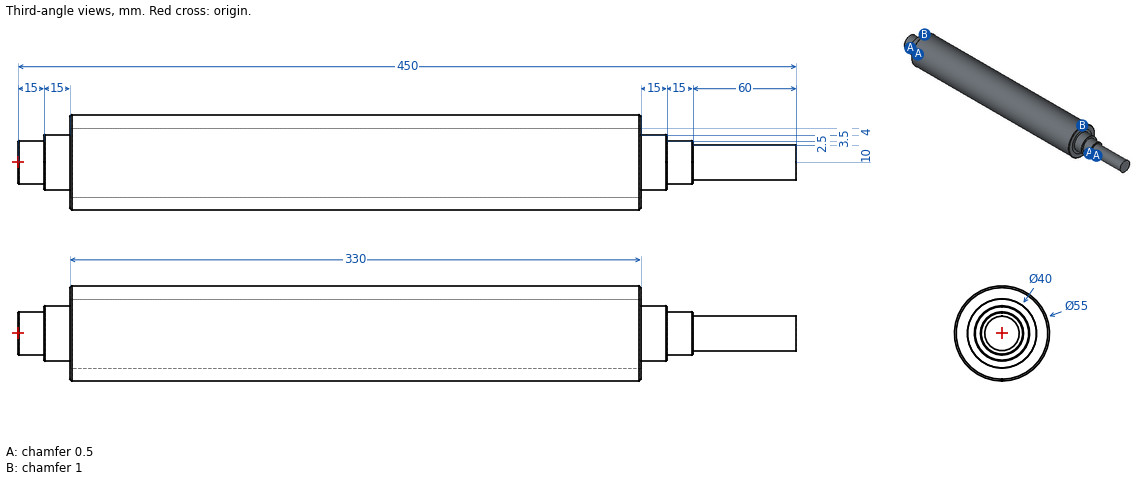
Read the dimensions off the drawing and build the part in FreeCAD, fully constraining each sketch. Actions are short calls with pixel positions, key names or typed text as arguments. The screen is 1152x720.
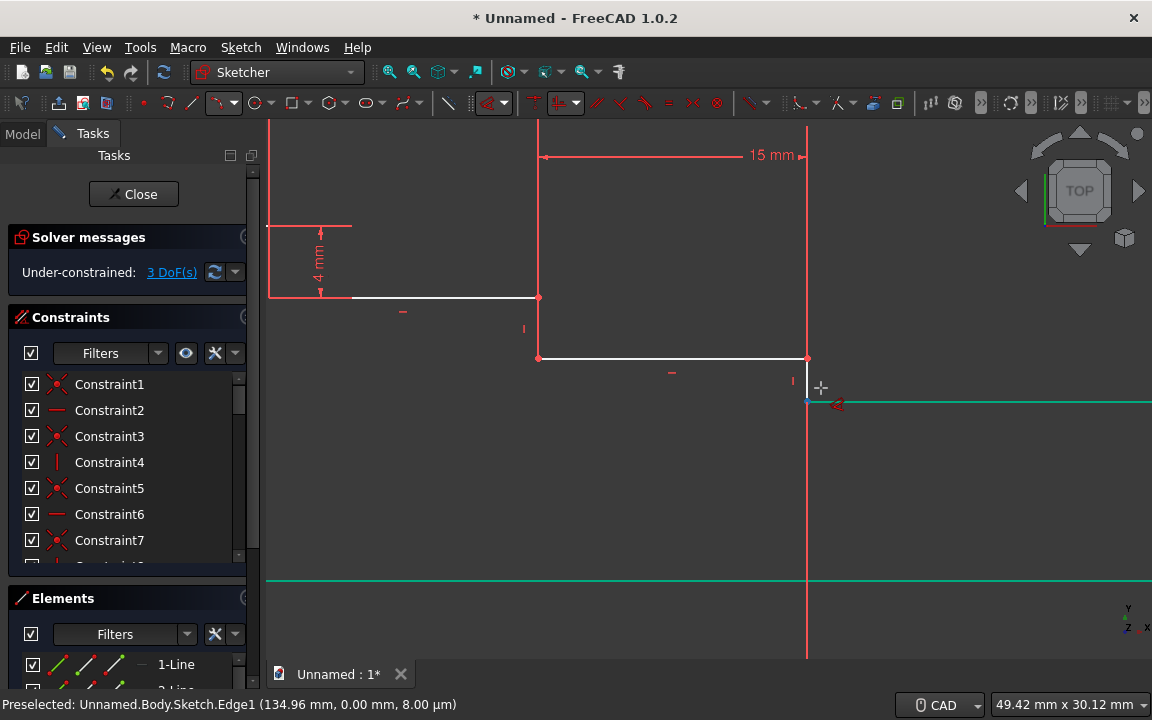
click(807, 380)
click(841, 380)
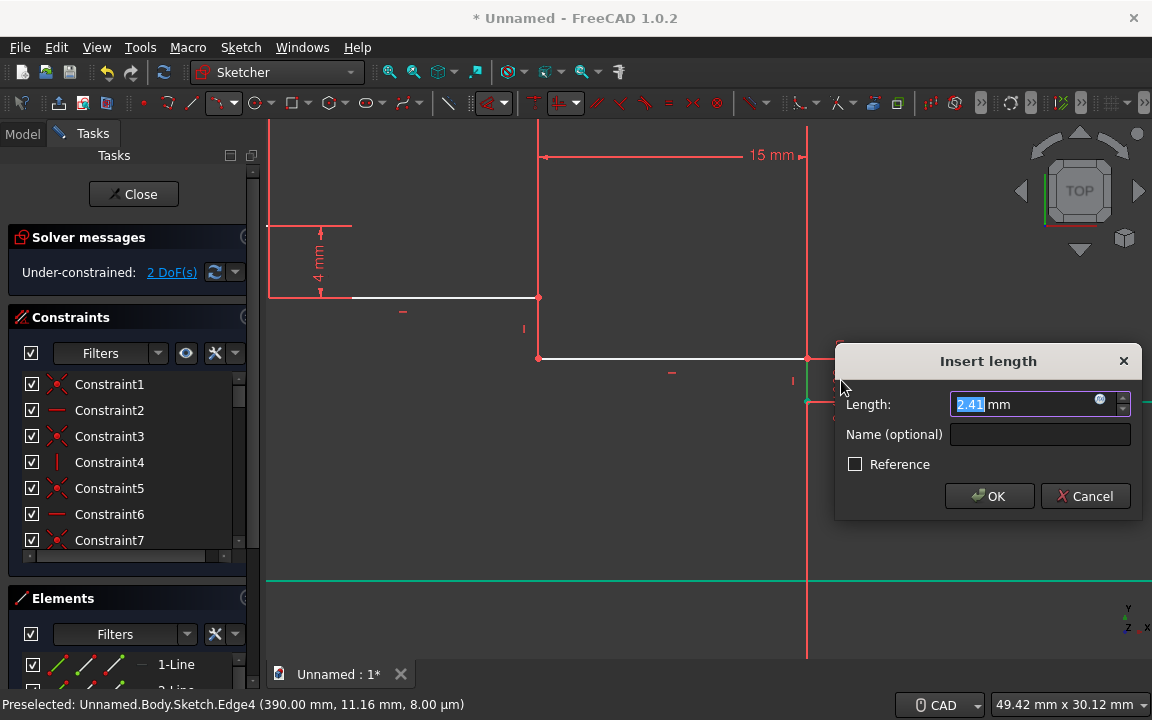
text(2.5)
key(Return)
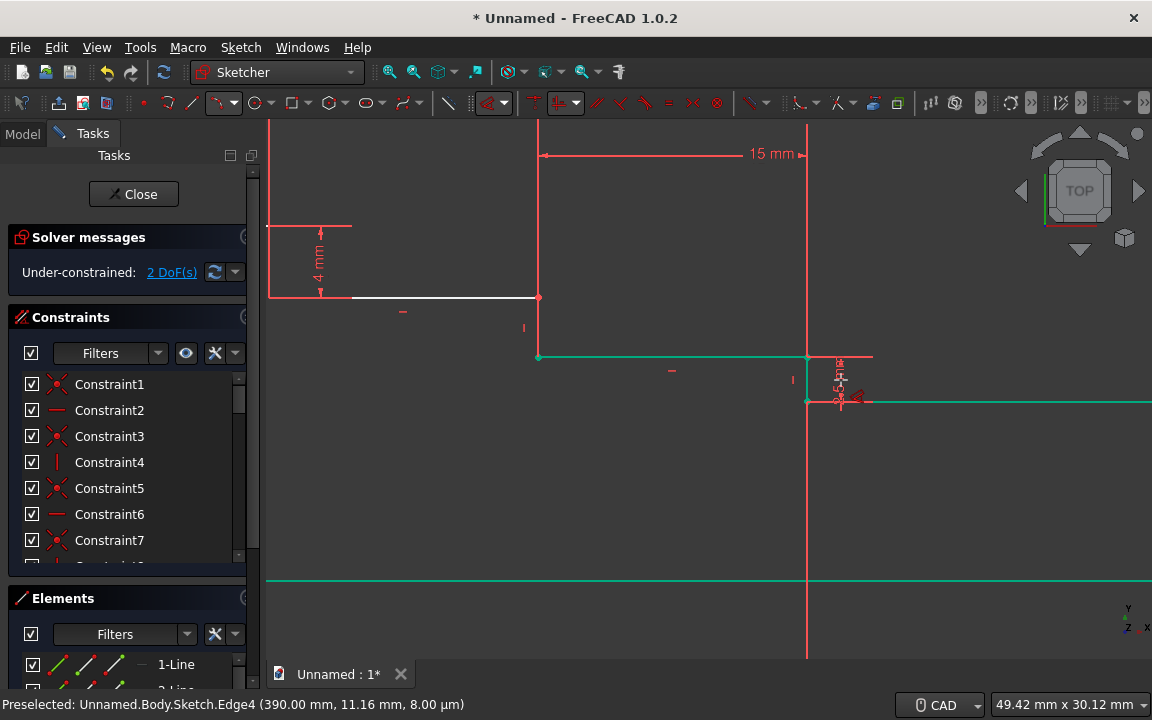
click(538, 339)
click(572, 327)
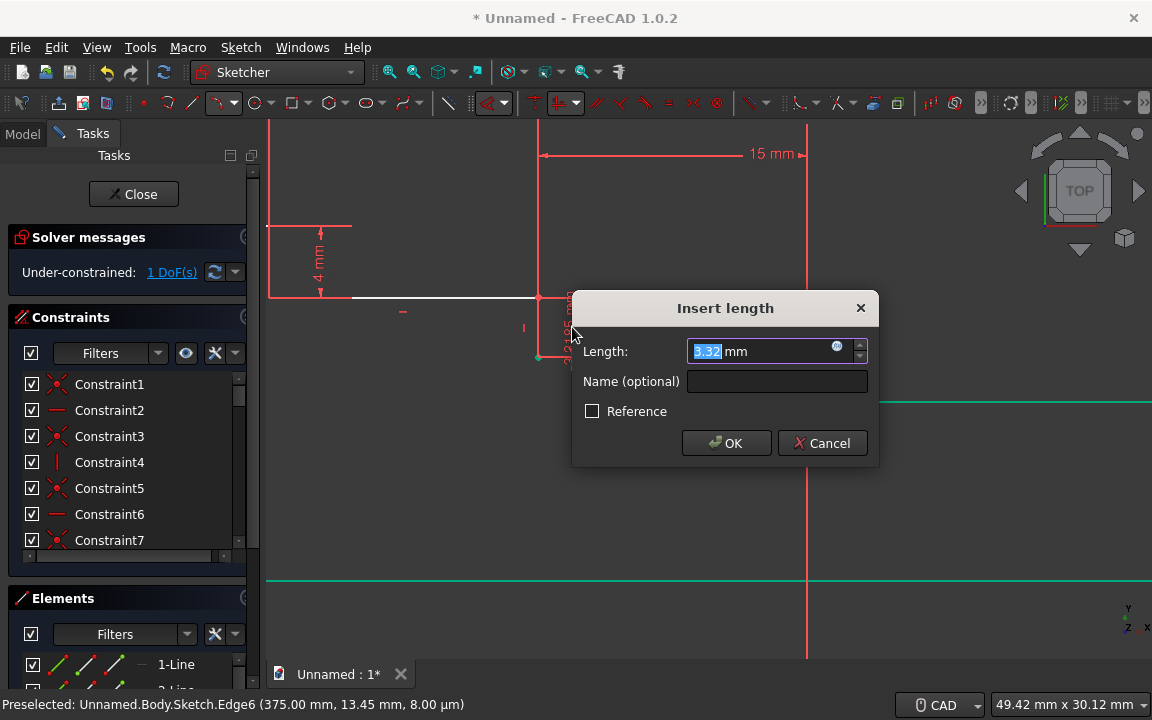
text(3.5)
key(Return)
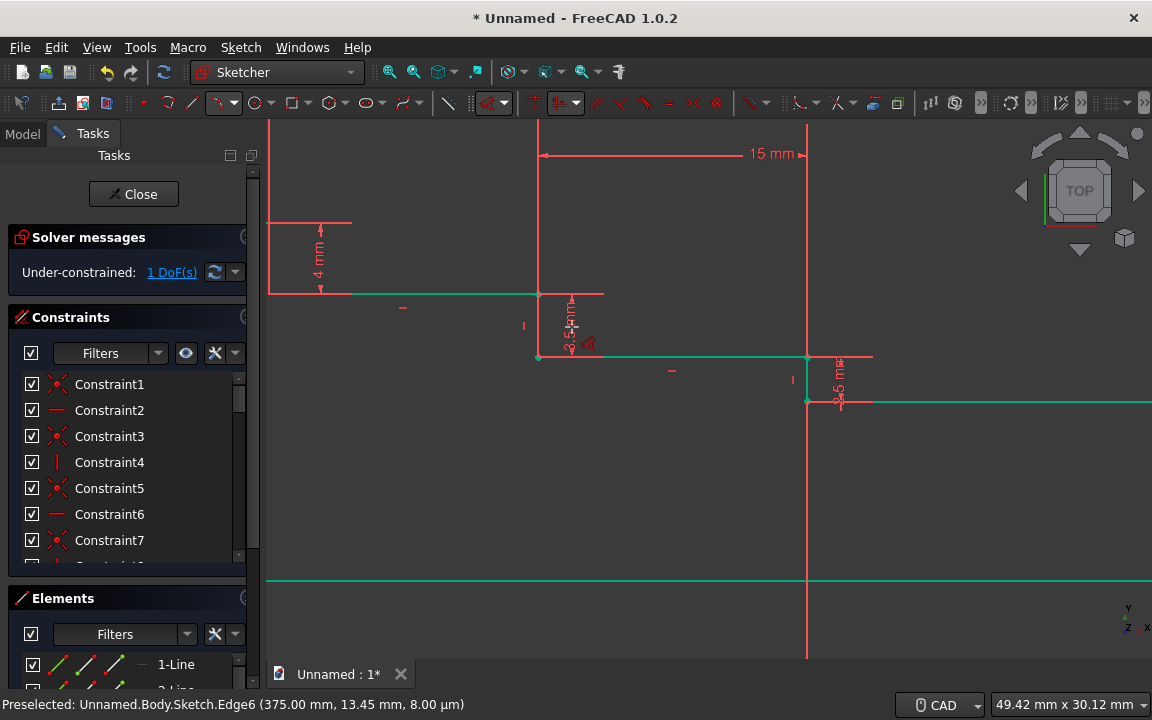
scroll(821, 388, down, 14)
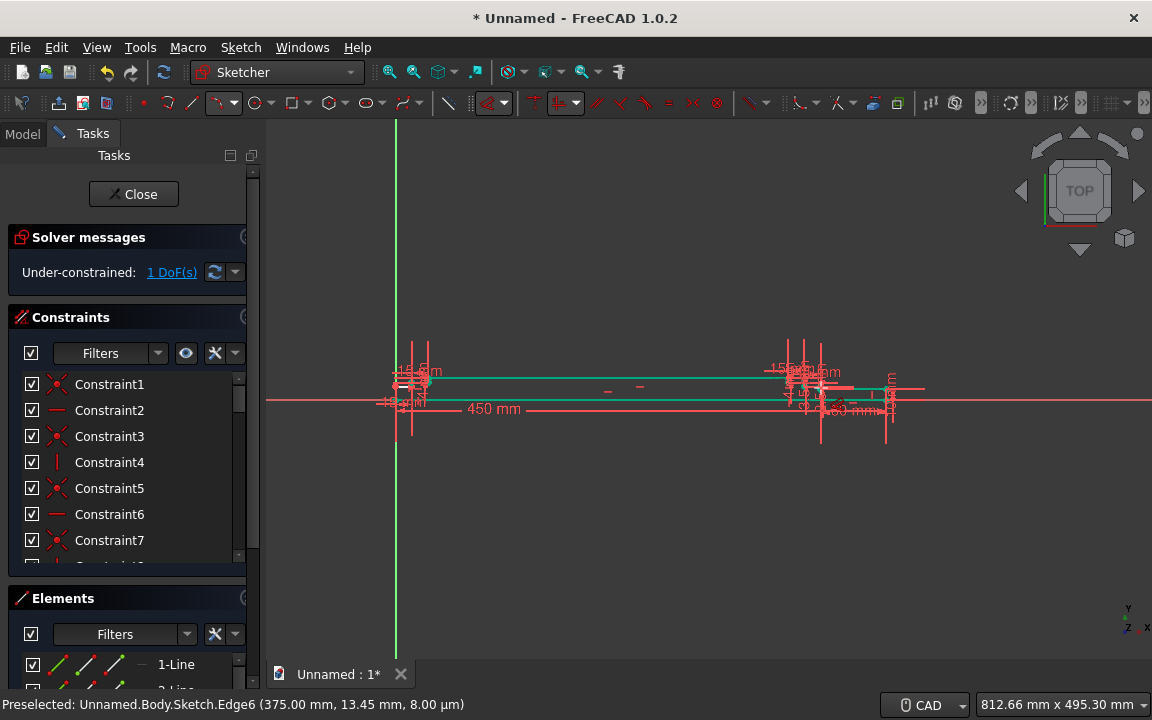
scroll(412, 384, up, 13)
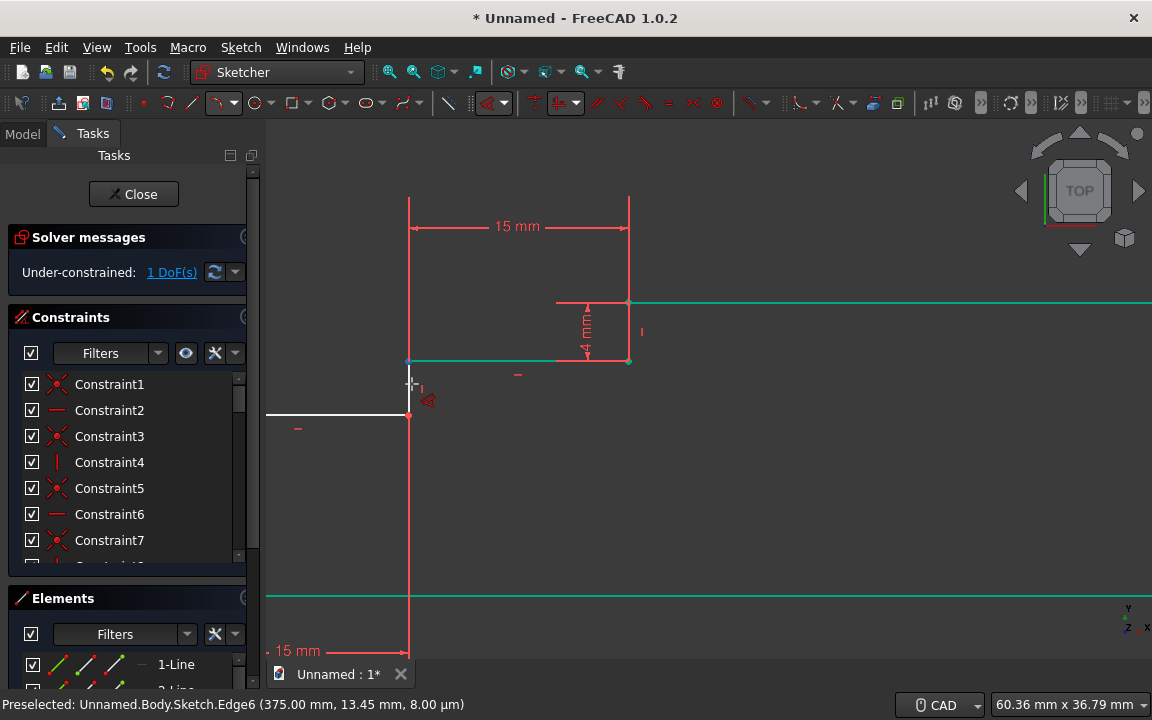
click(409, 378)
click(375, 388)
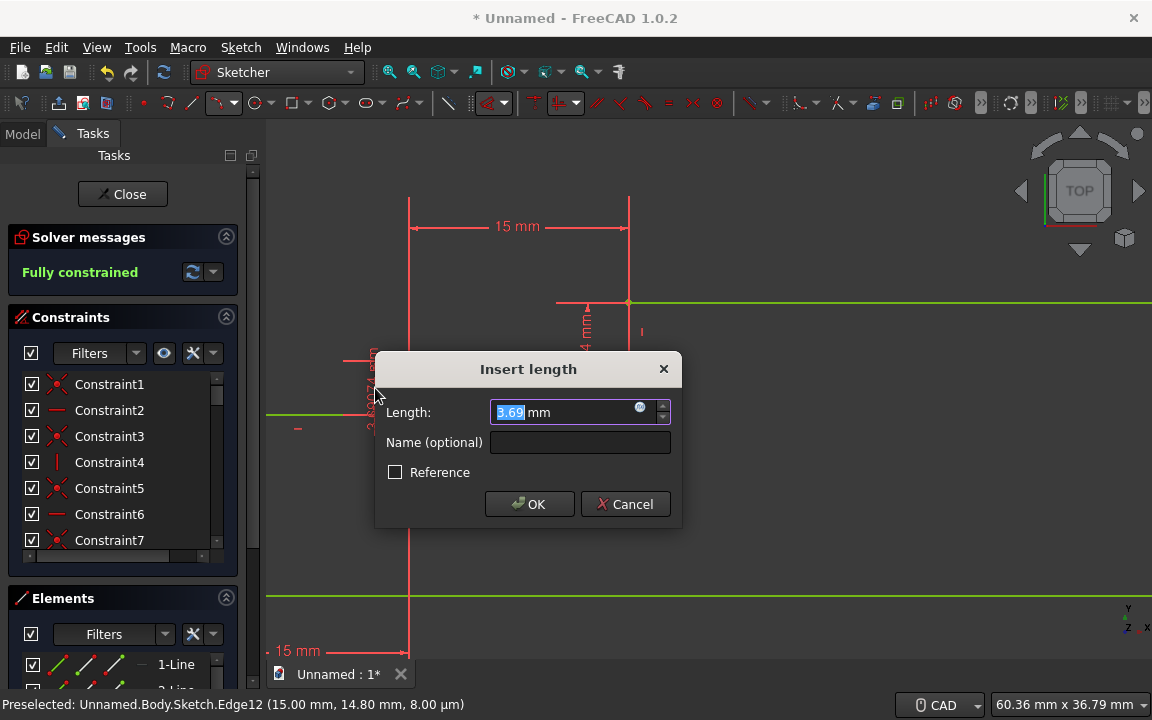
text(3.5)
key(Return)
key(Escape)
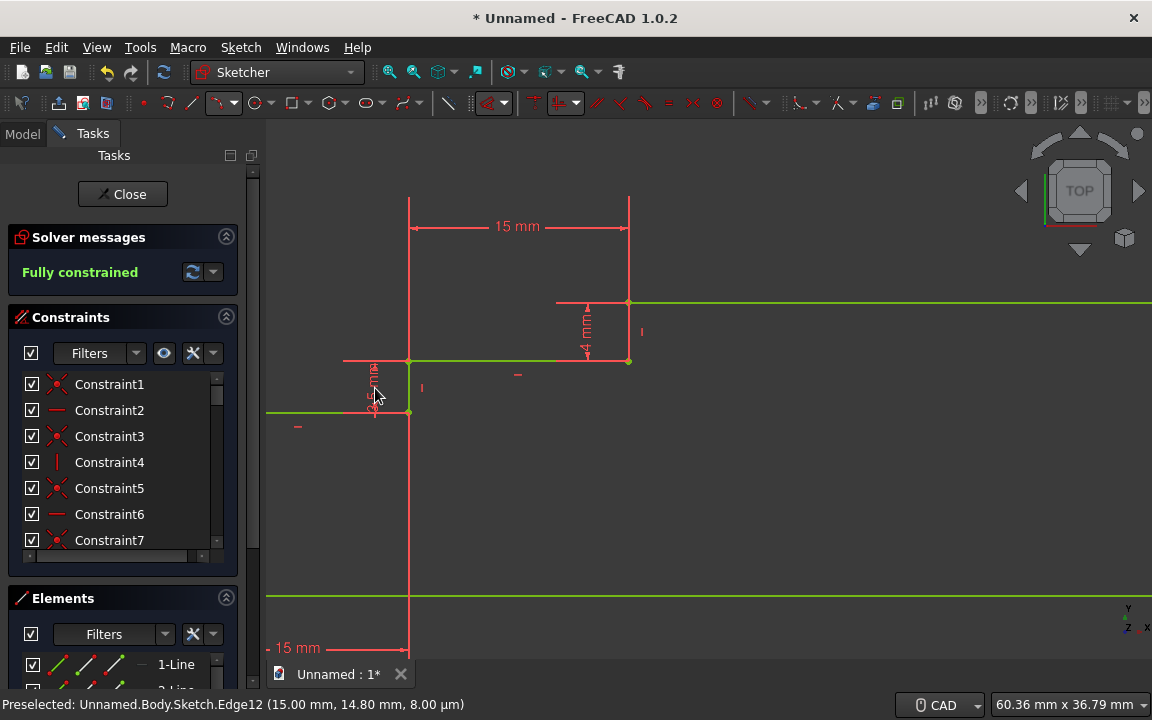
click(123, 194)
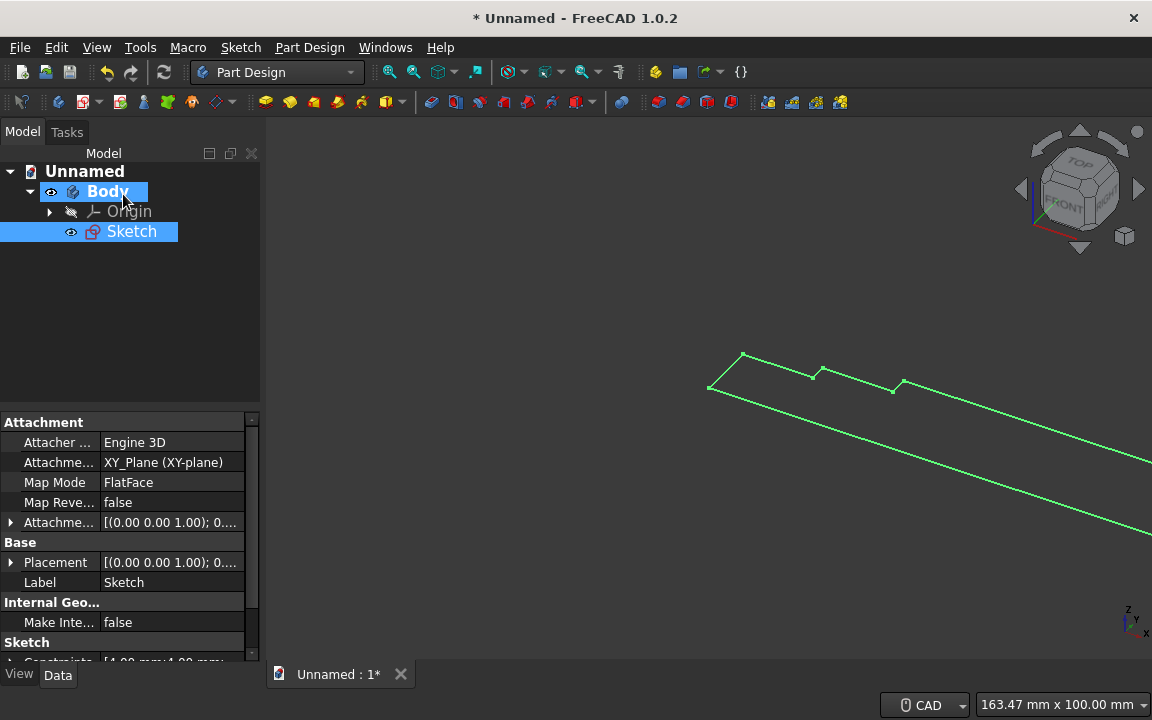
click(290, 102)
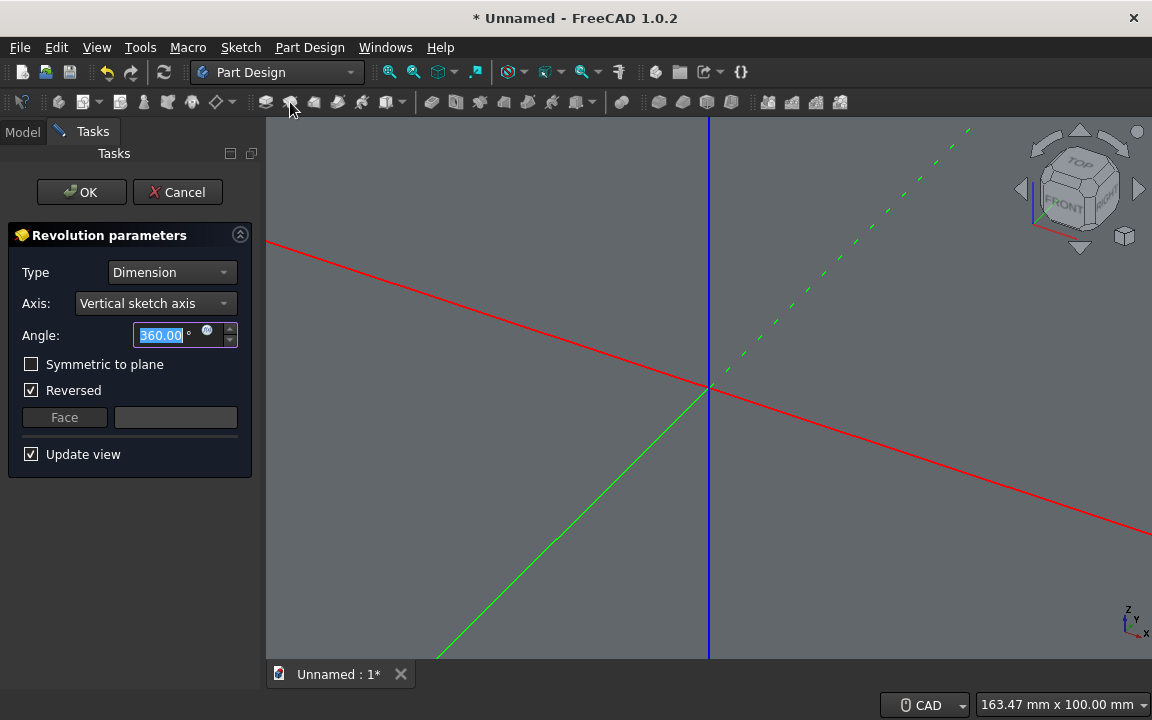
click(156, 304)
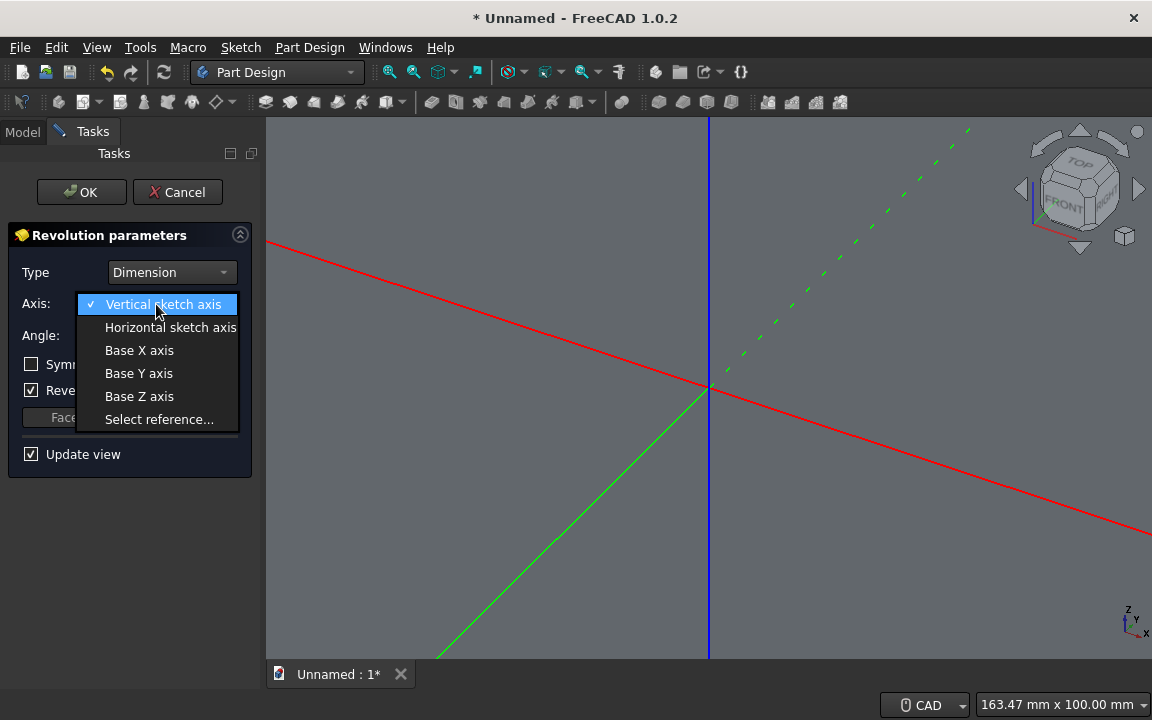
click(156, 328)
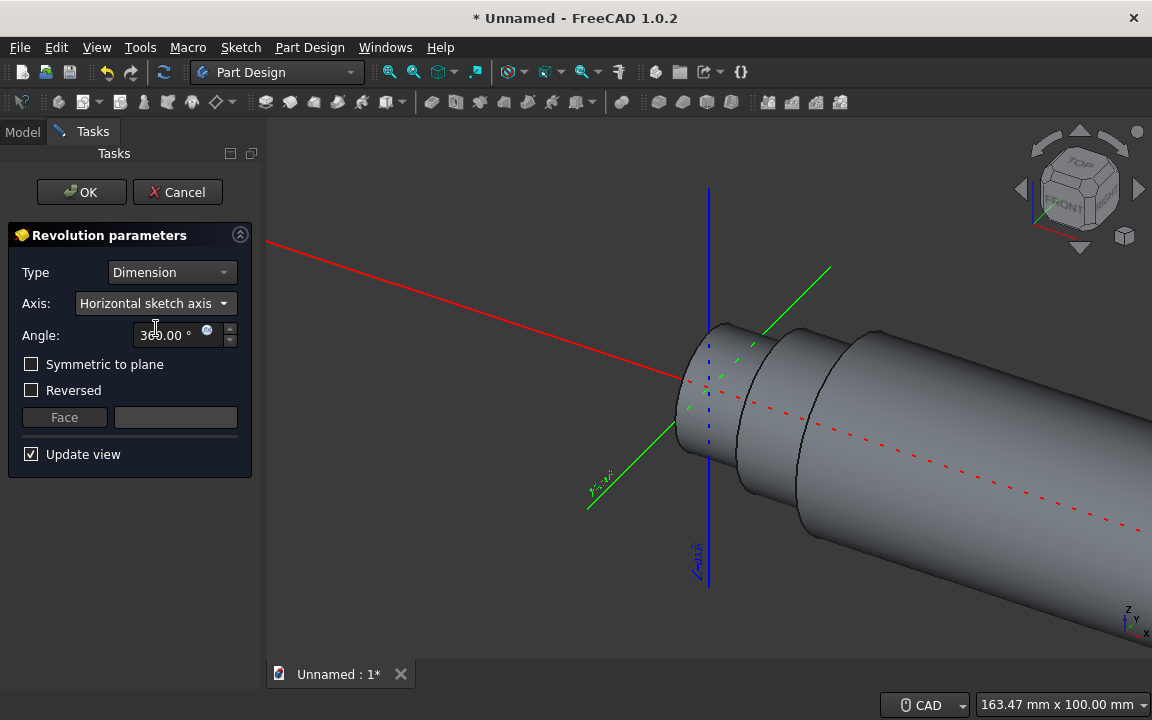
click(82, 192)